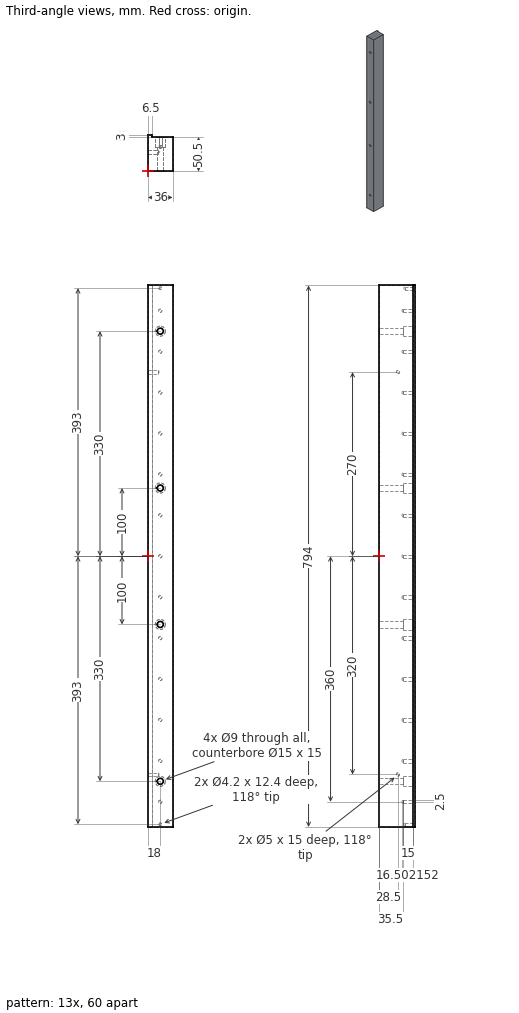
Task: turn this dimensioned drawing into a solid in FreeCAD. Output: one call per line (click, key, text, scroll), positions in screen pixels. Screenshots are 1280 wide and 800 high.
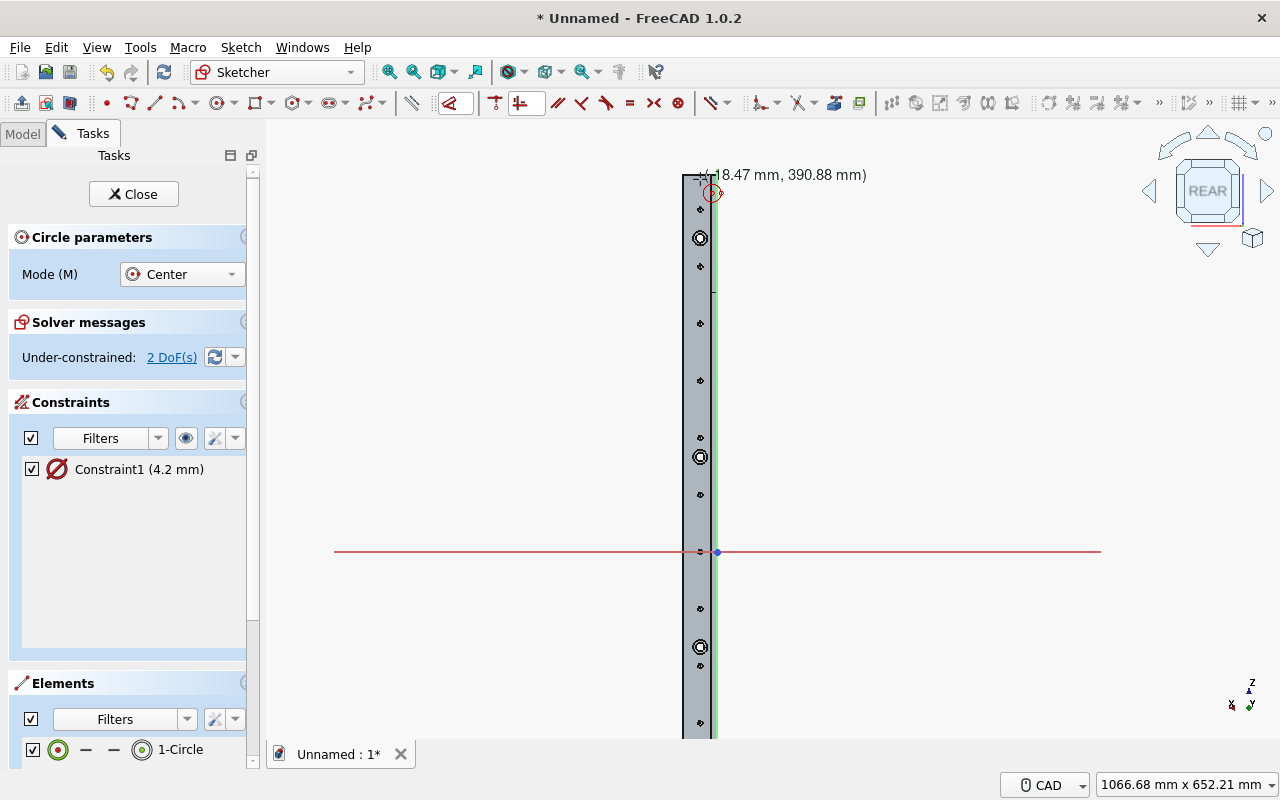
click(700, 178)
move(702, 177)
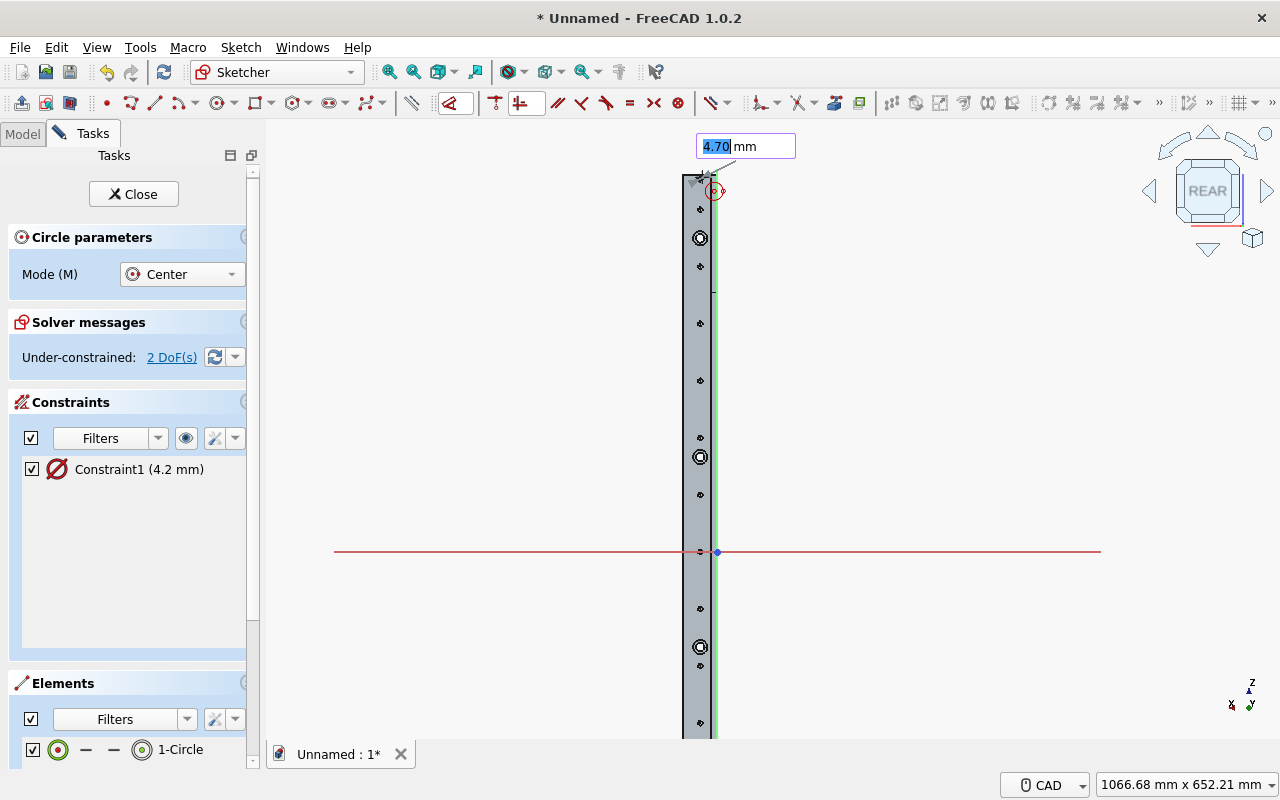
text(4.2)
key(Return)
key(Escape)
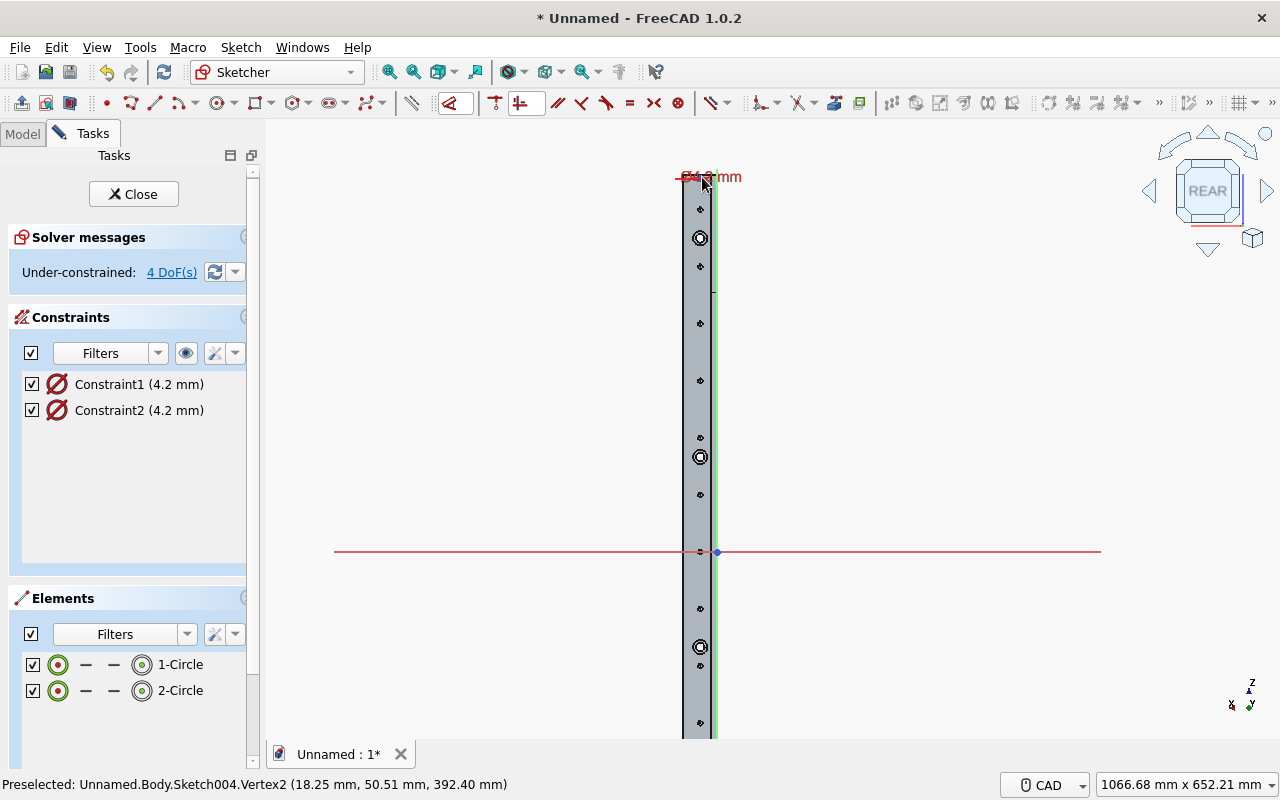
scroll(700, 279, down, 3)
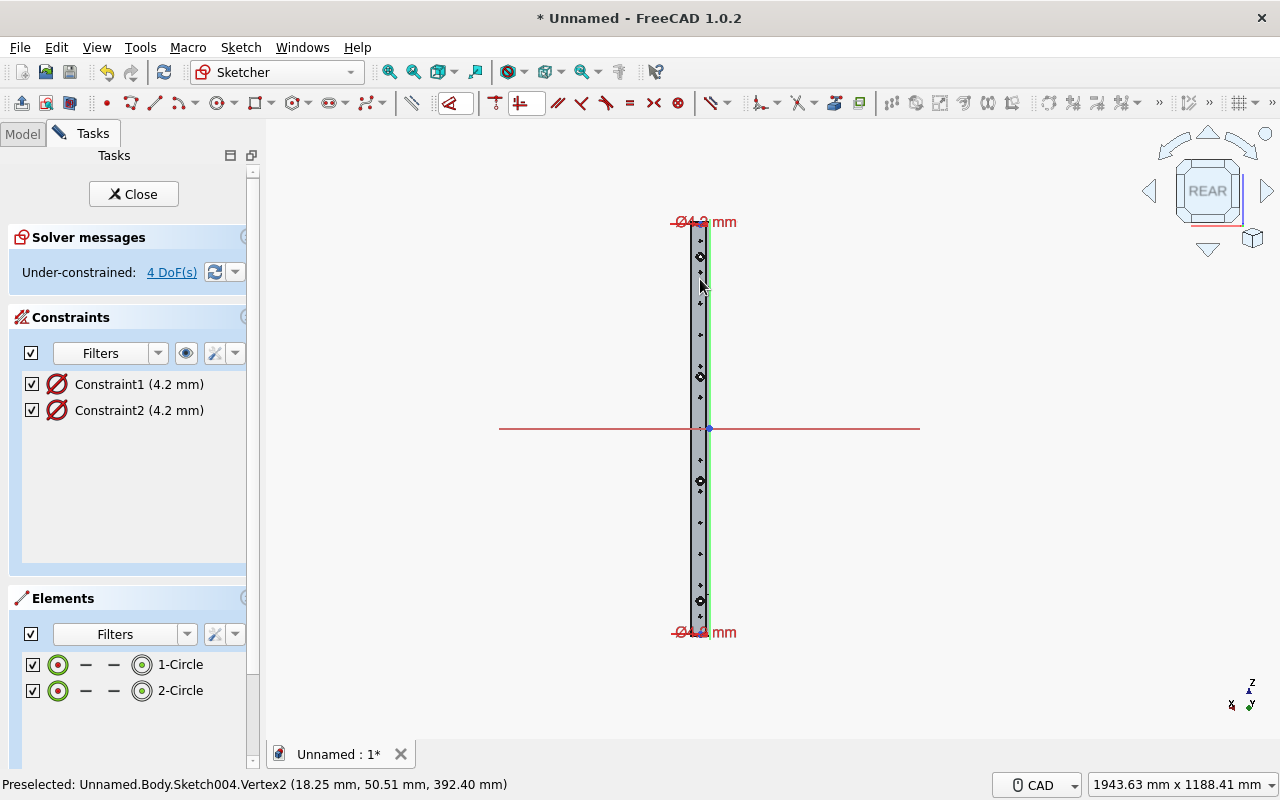
click(700, 634)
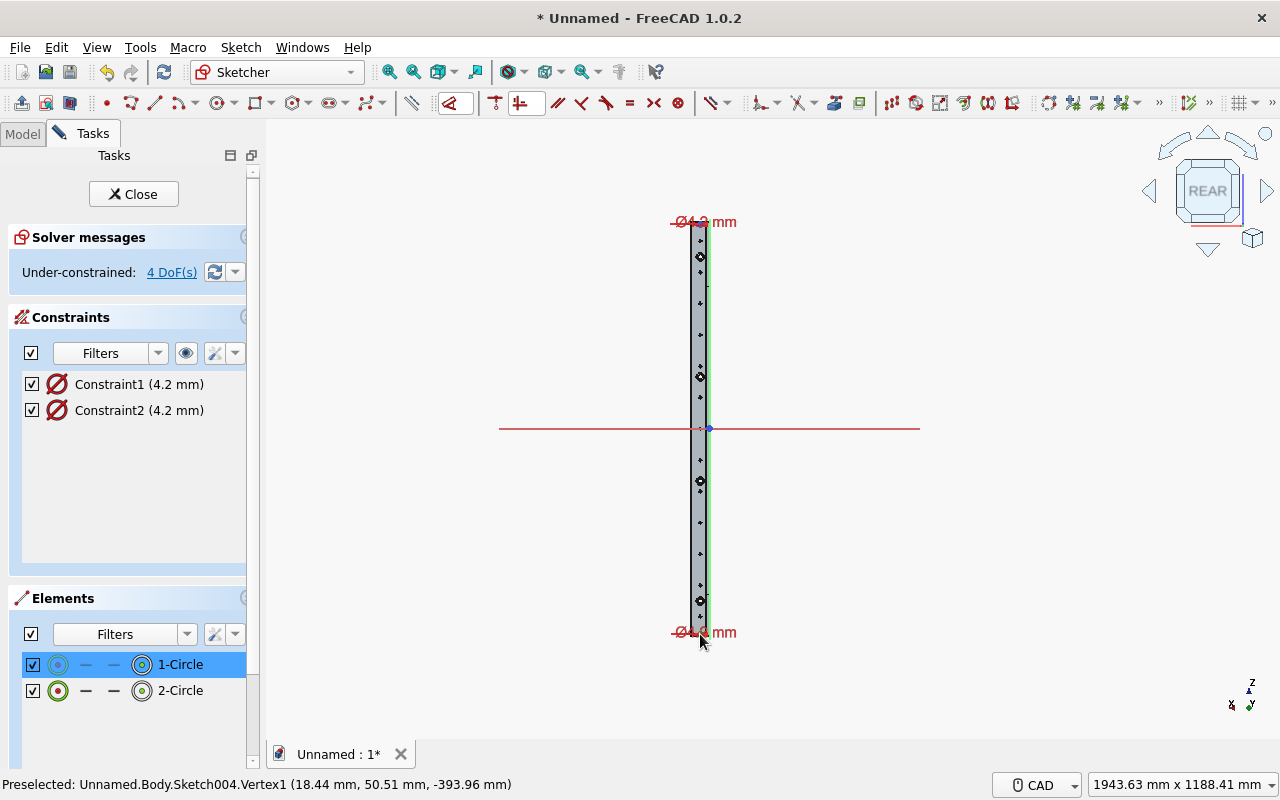
click(700, 224)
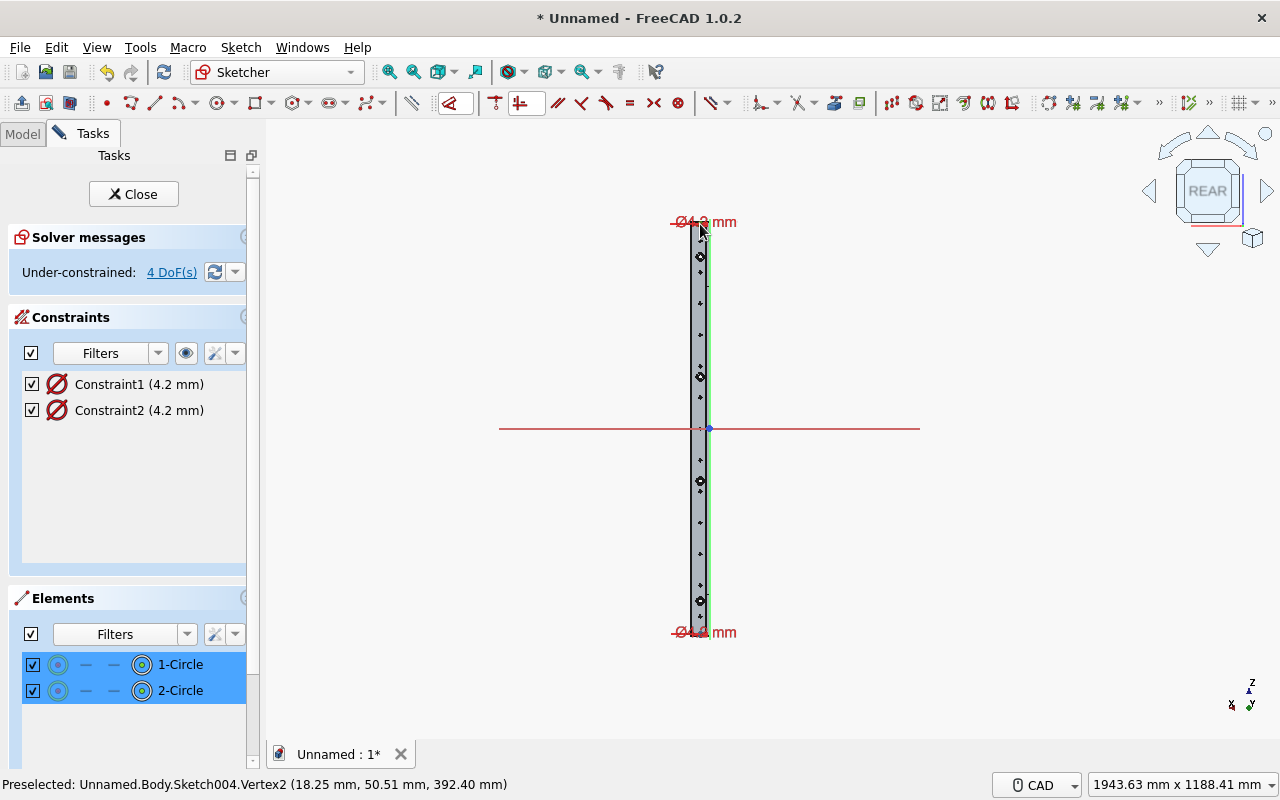
click(540, 104)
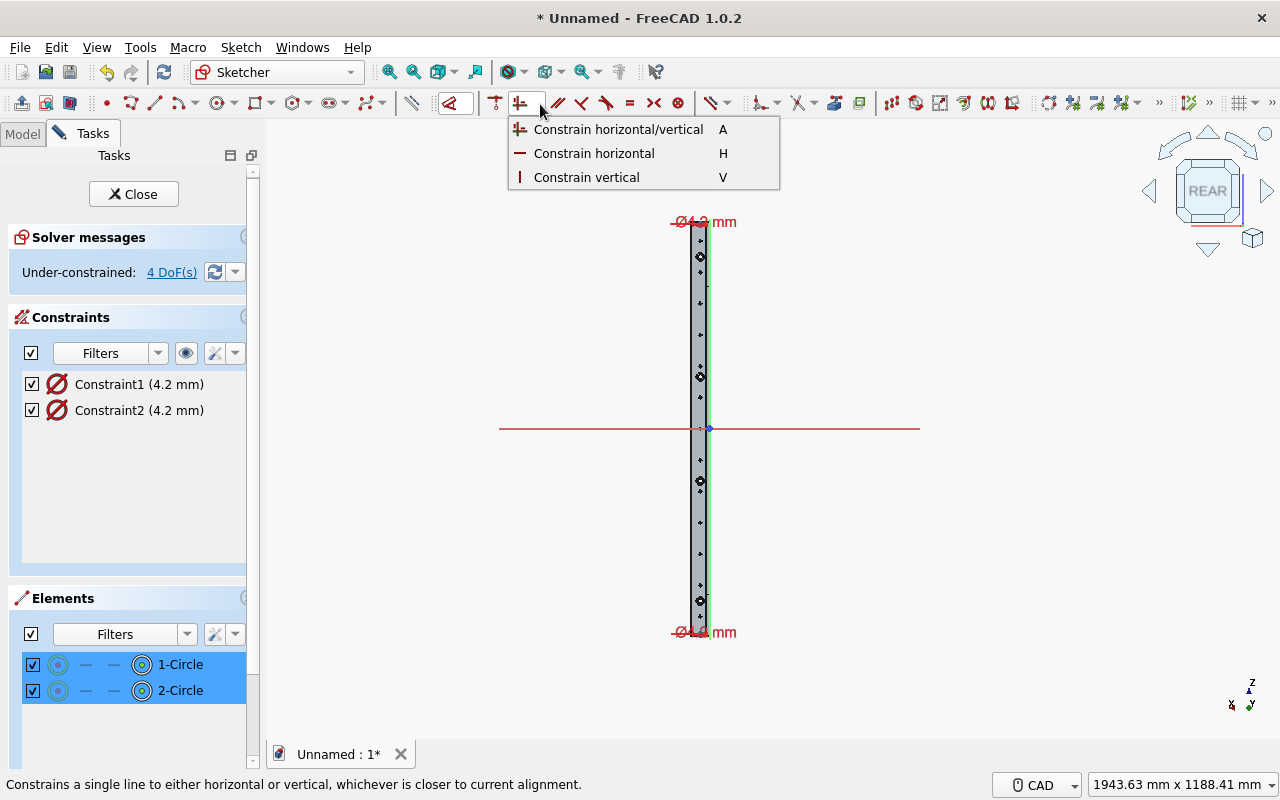
click(644, 177)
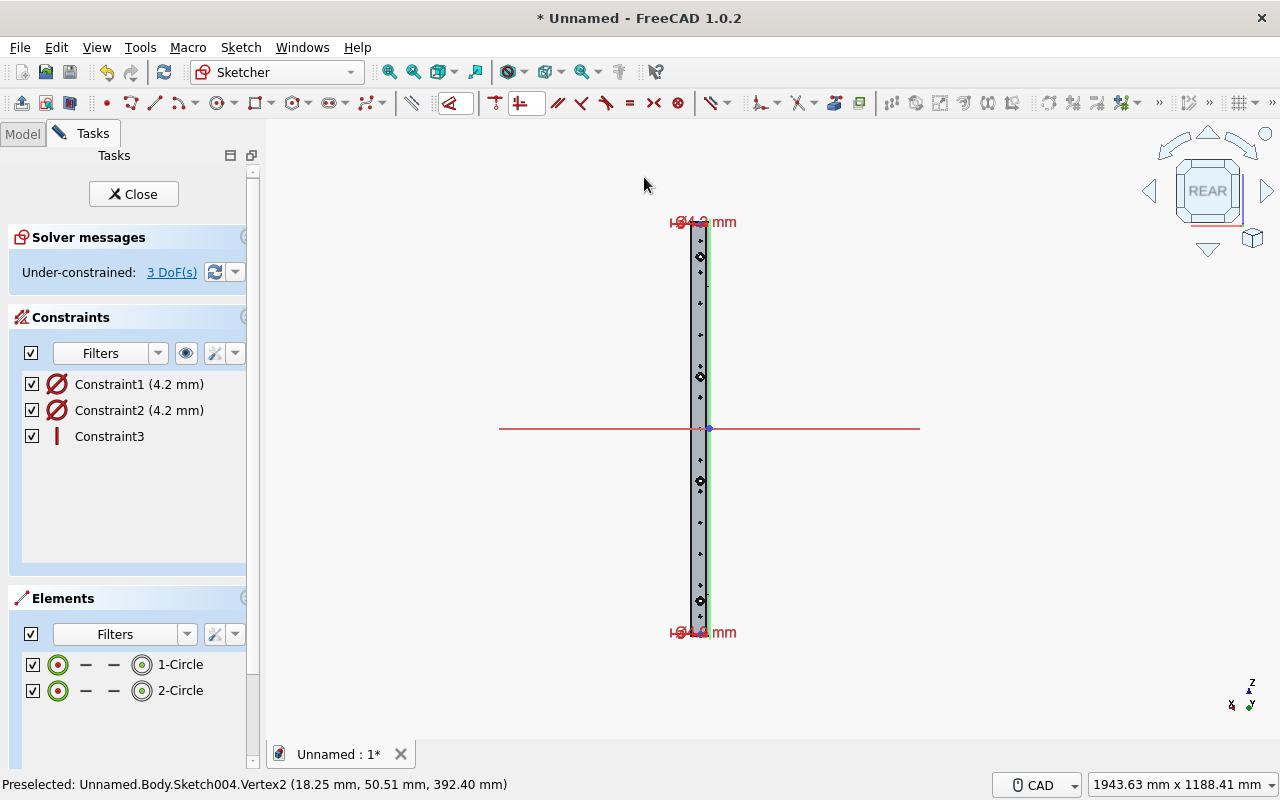
scroll(700, 634, up, 8)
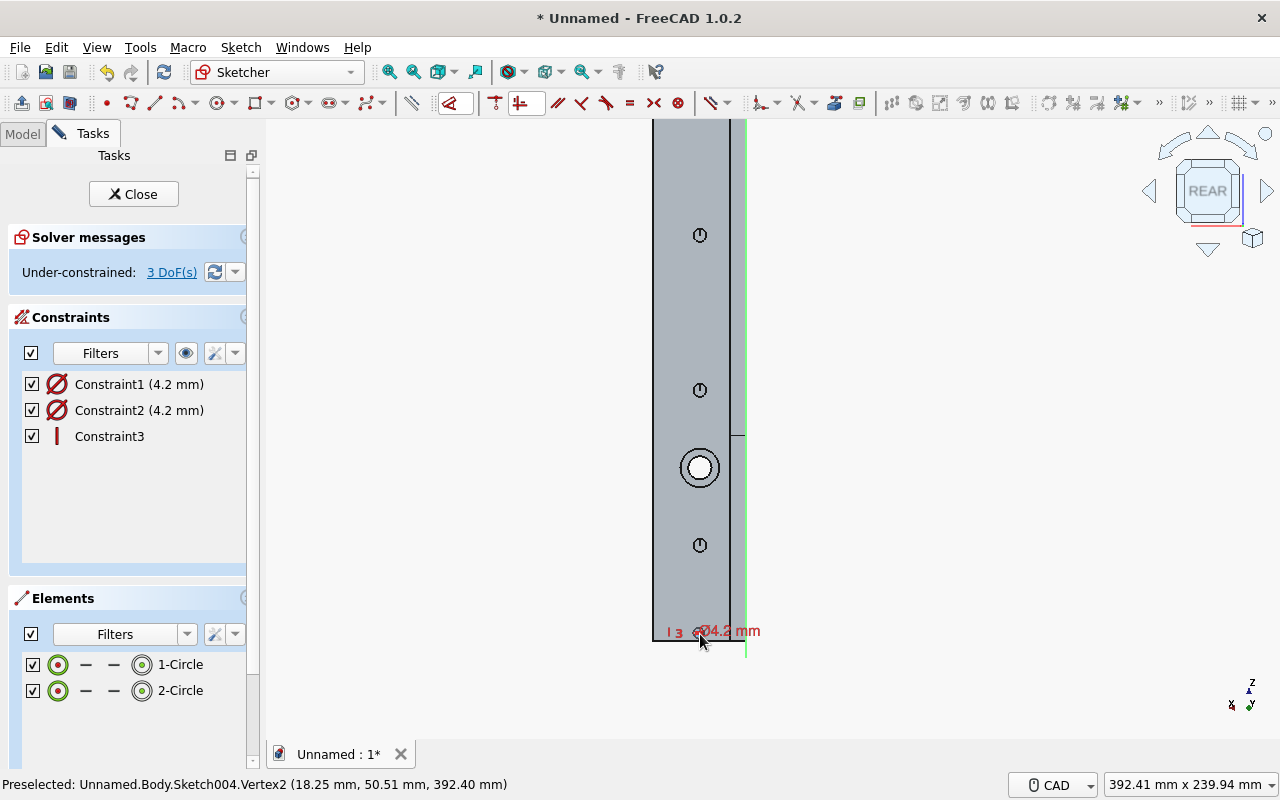
click(699, 633)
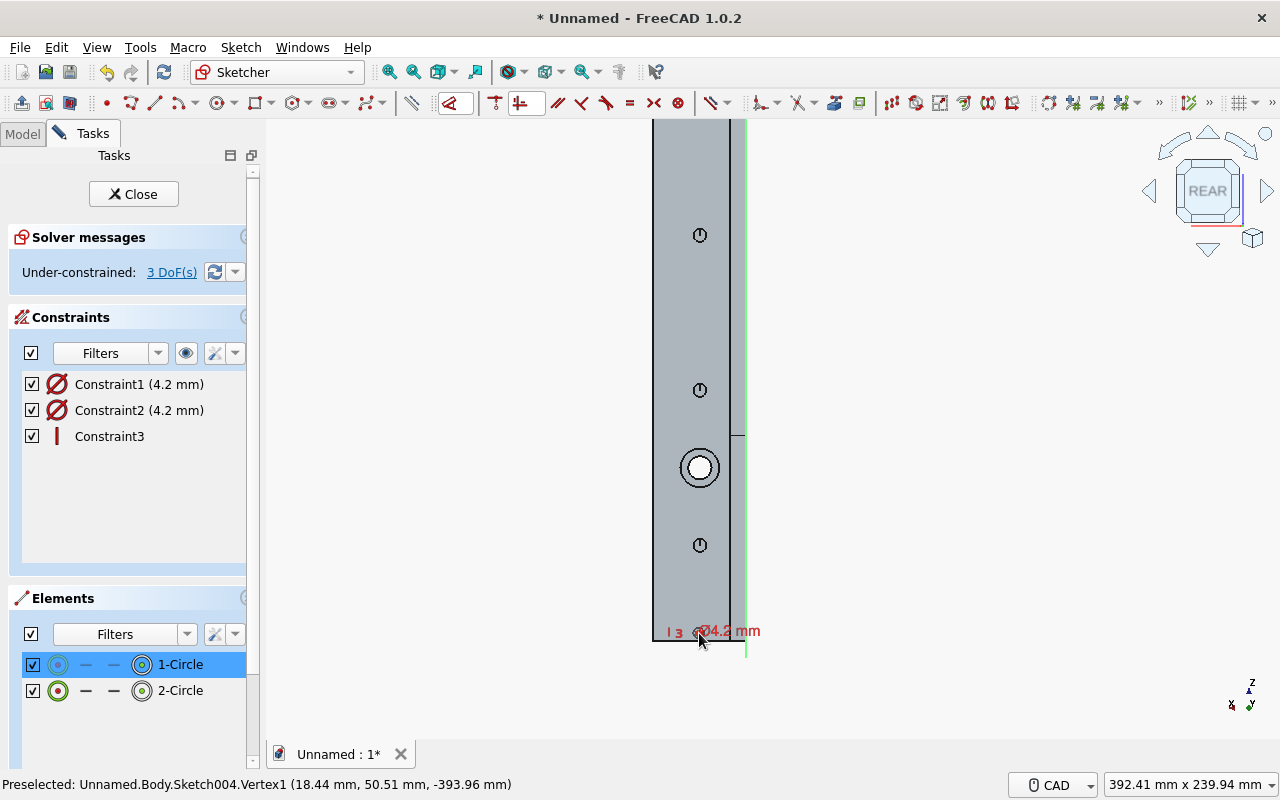
key(l)